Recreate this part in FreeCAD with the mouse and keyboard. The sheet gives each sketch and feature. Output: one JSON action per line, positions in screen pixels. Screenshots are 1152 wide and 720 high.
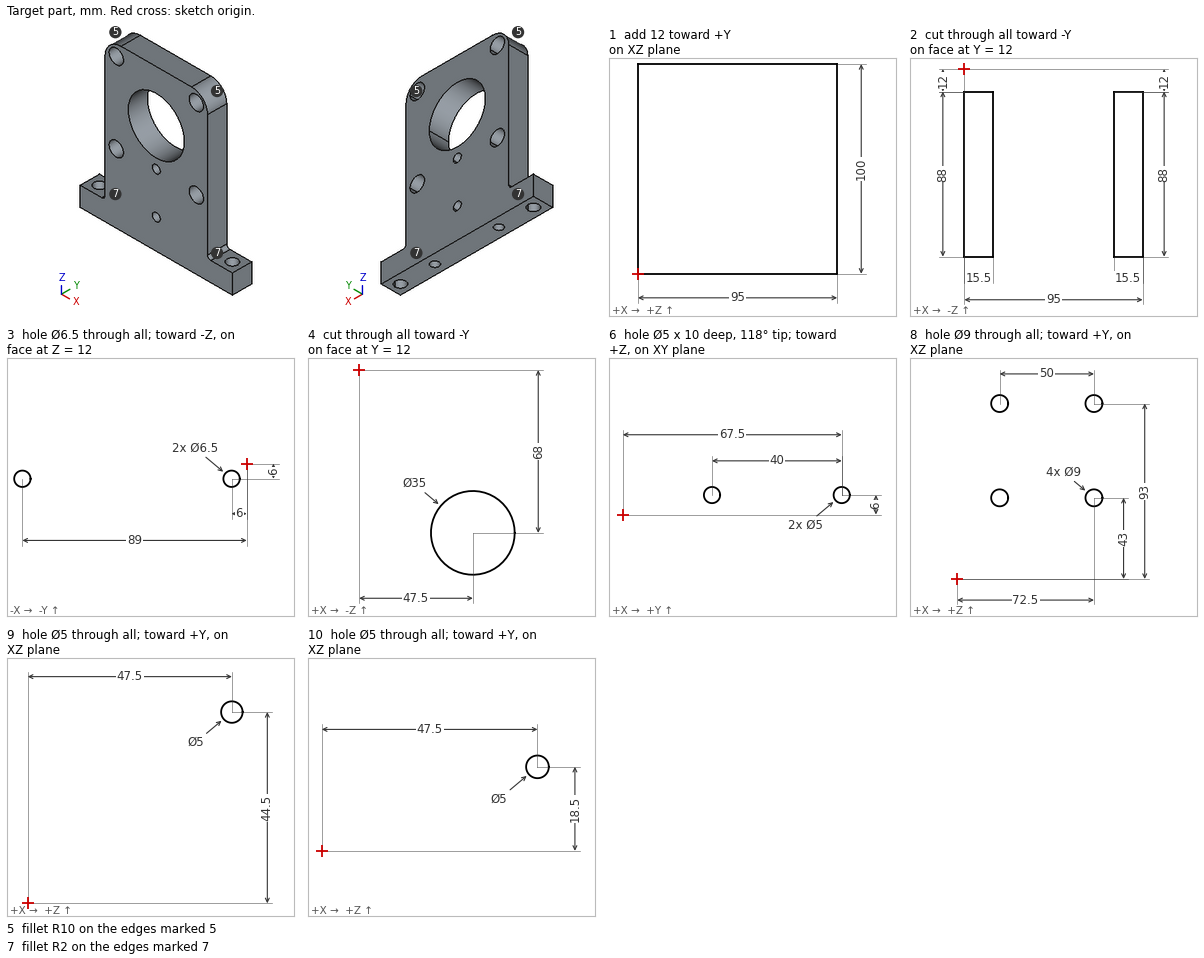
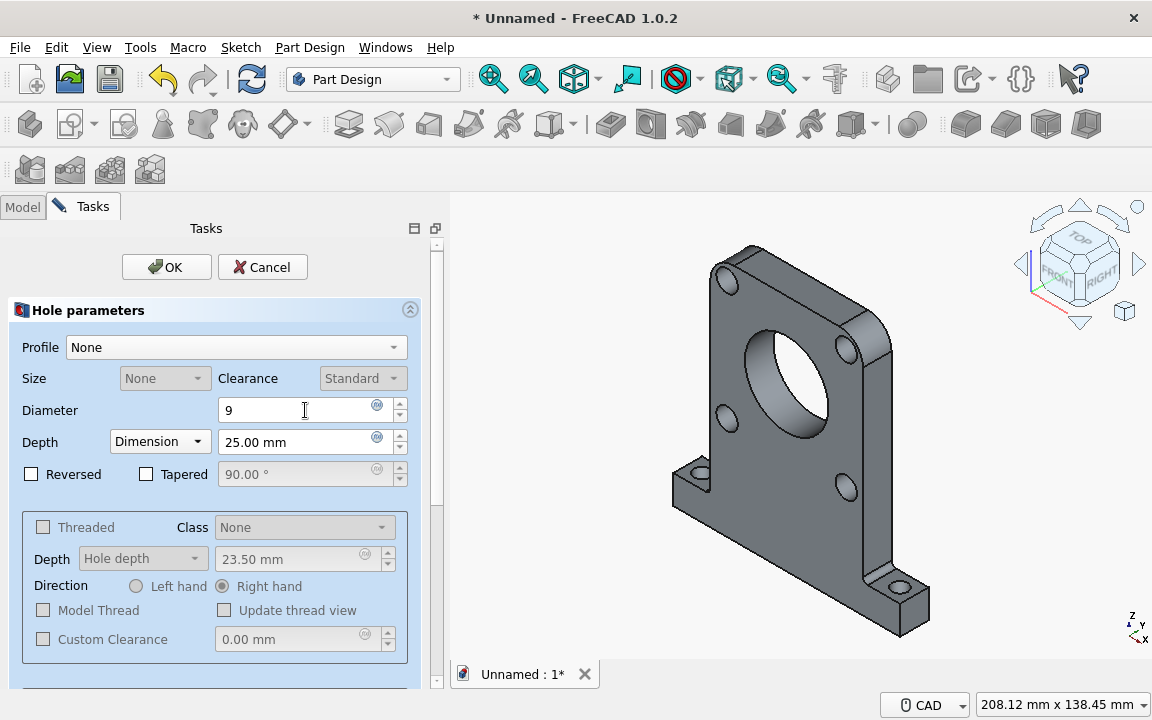
{"action": "left_click", "coordinate": [161, 442]}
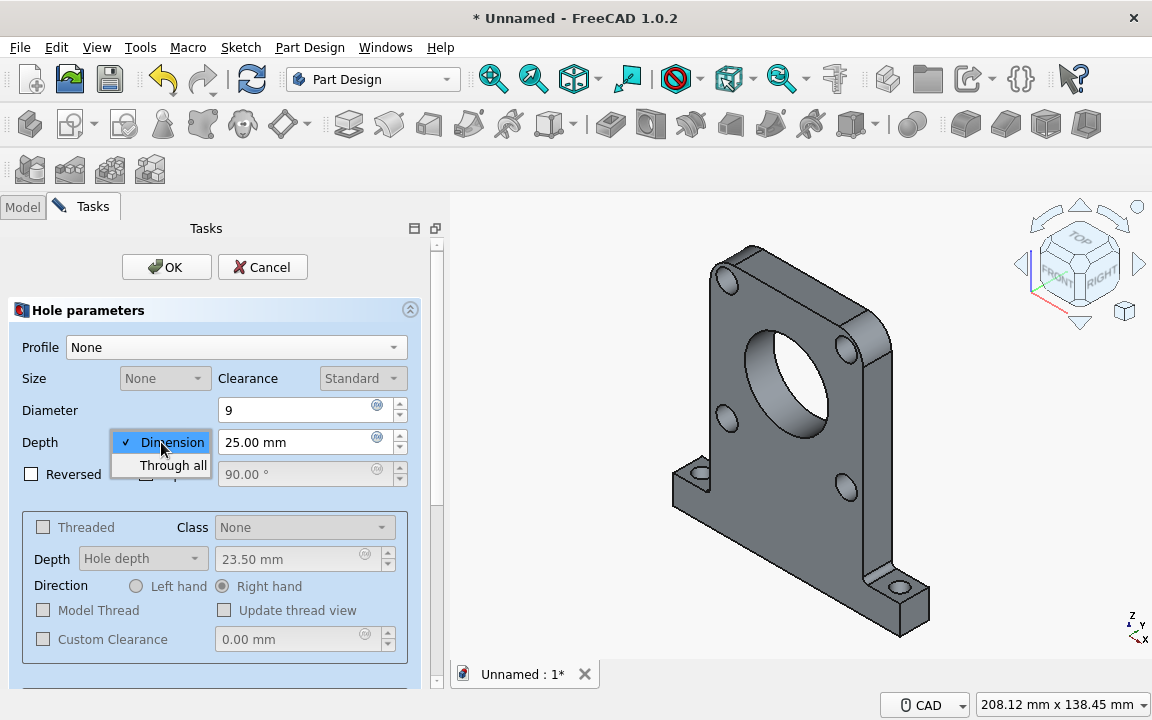
{"action": "left_click", "coordinate": [160, 466]}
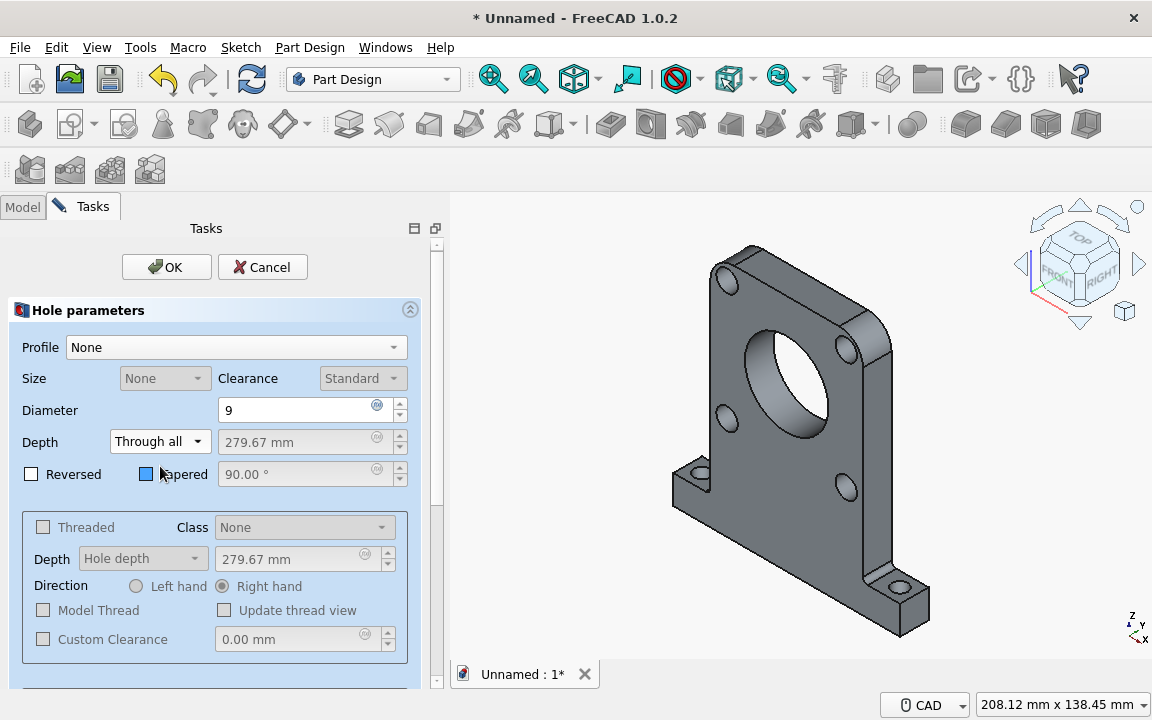
{"action": "left_click", "coordinate": [167, 267]}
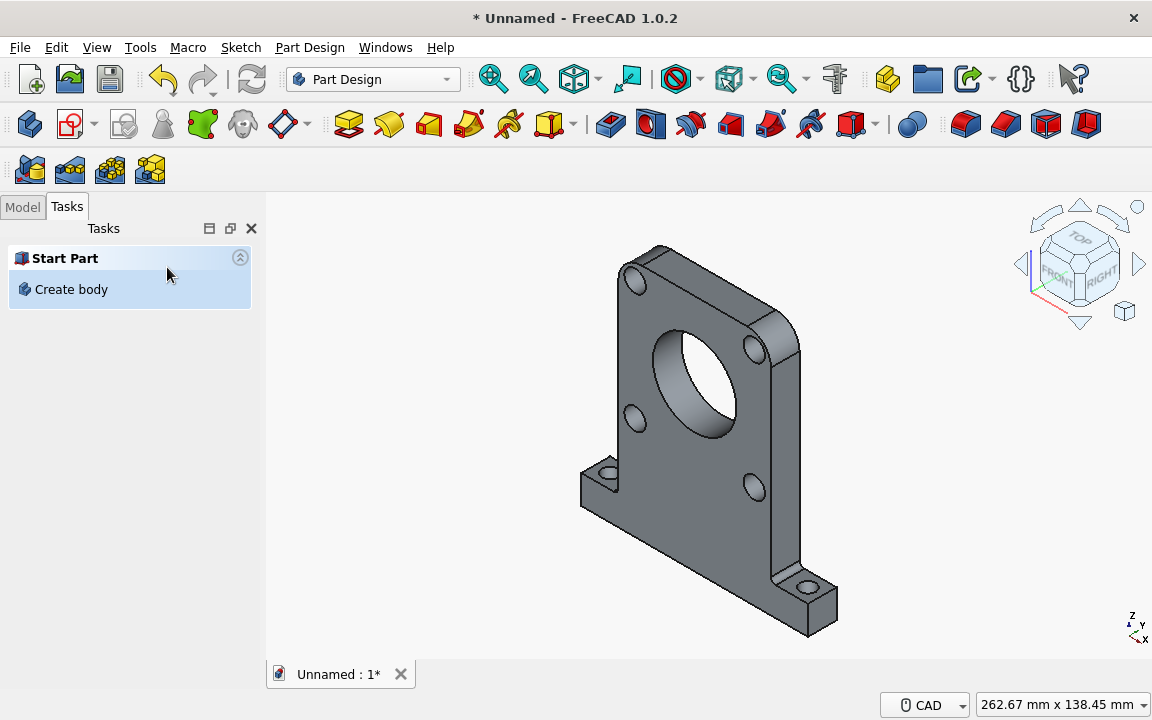
{"action": "left_click", "coordinate": [70, 124]}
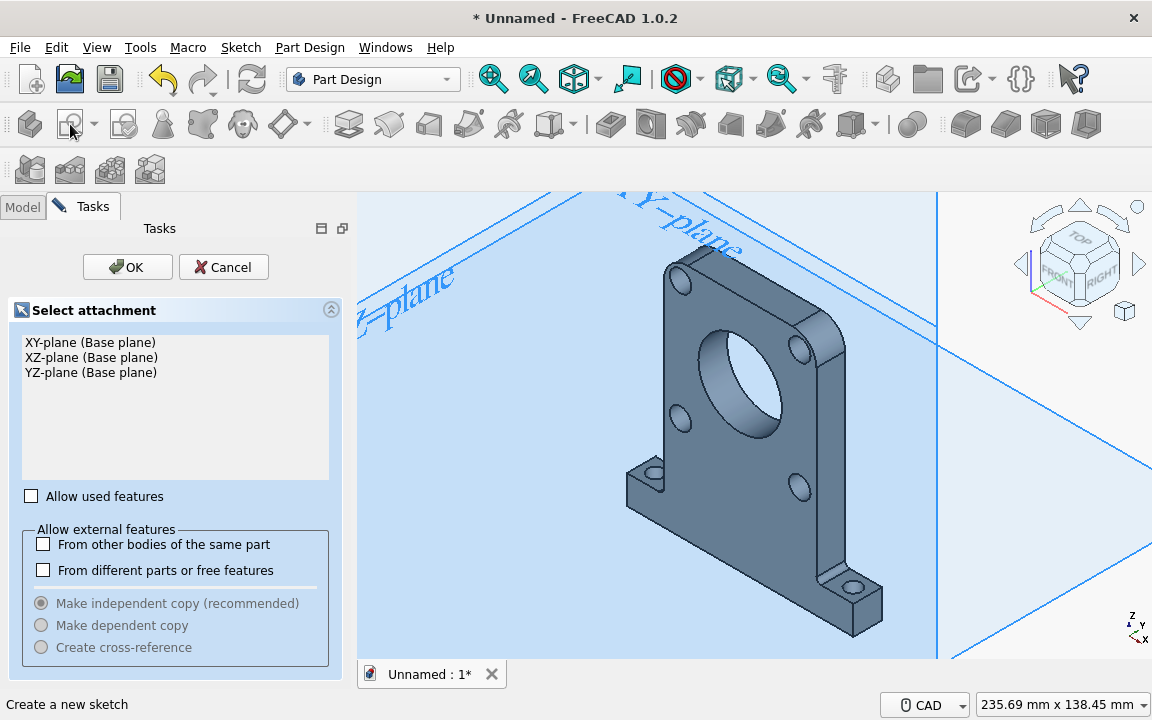
{"action": "left_click", "coordinate": [82, 358]}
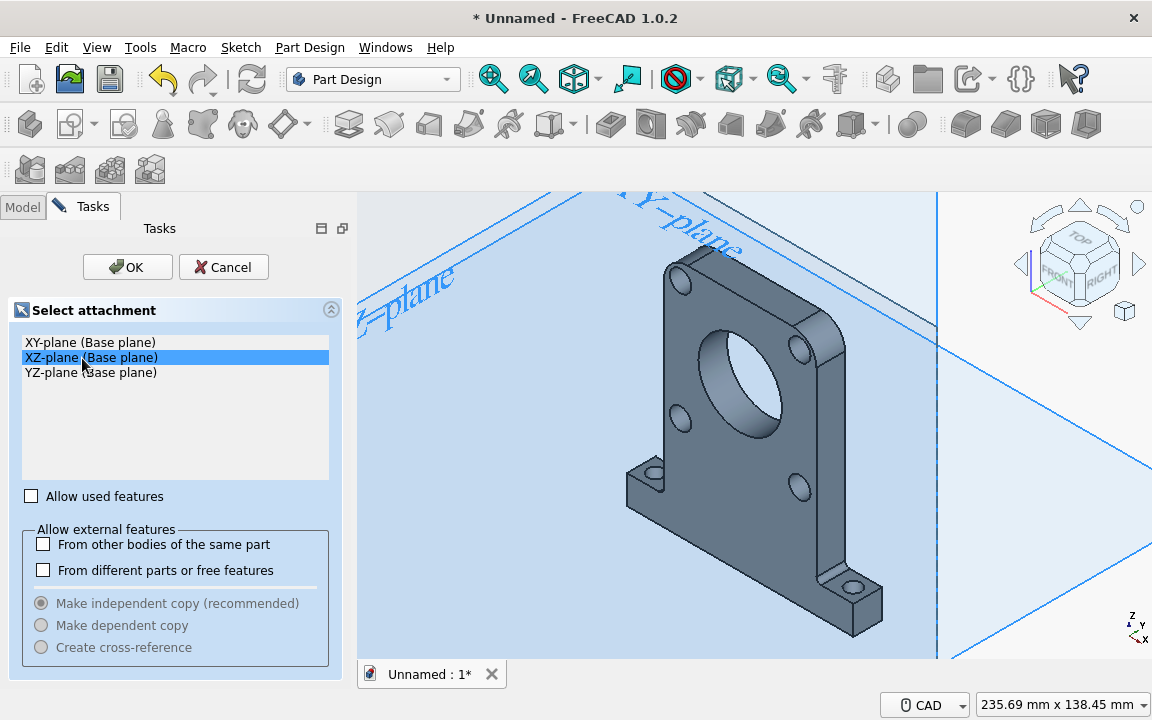
{"action": "left_click", "coordinate": [128, 267]}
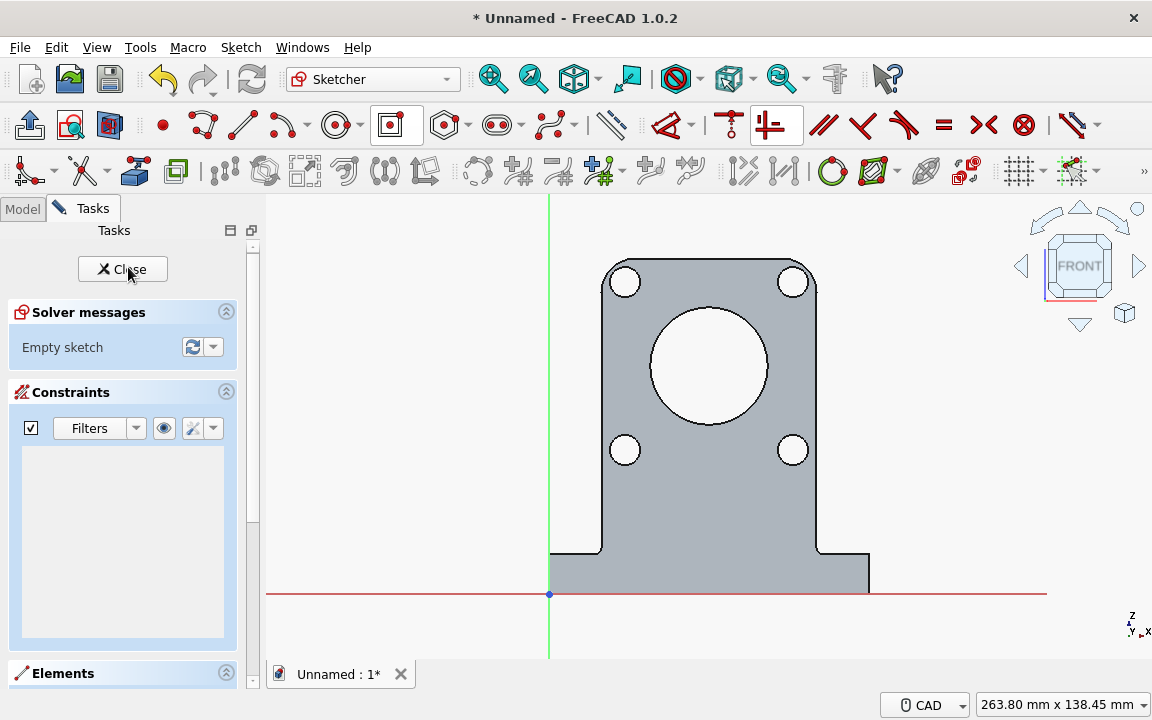
{"action": "scroll", "coordinate": [713, 446], "scroll_direction": "up", "scroll_amount": 14}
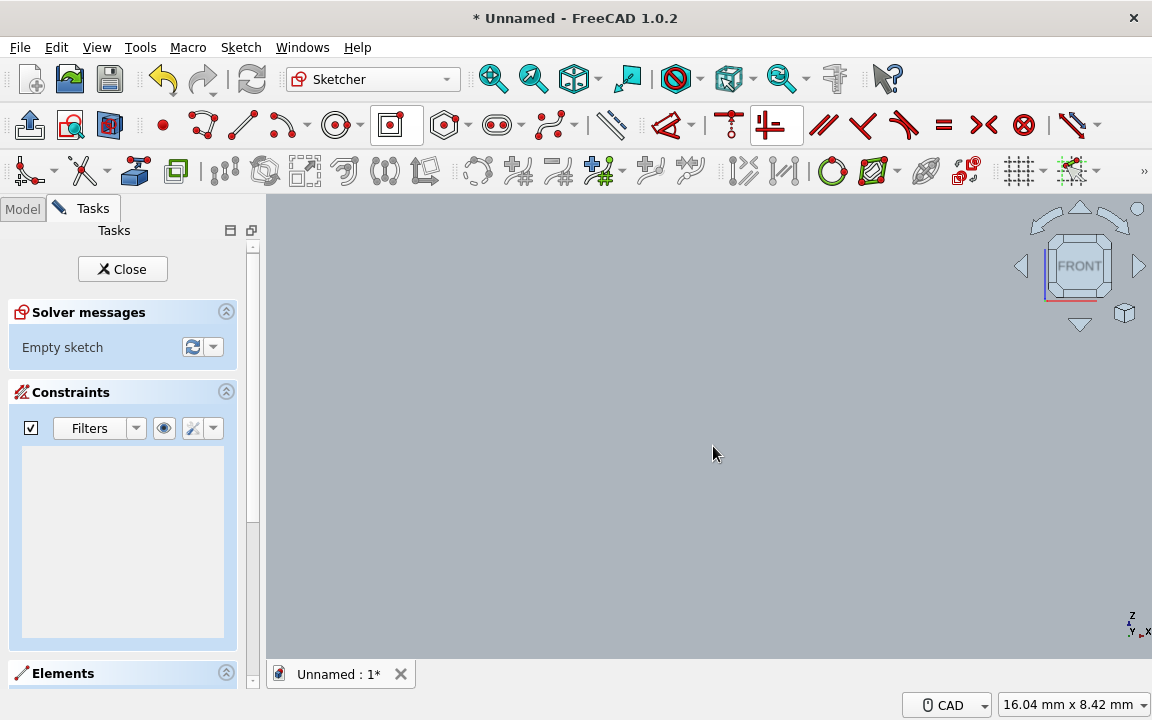
{"action": "left_click", "coordinate": [336, 126]}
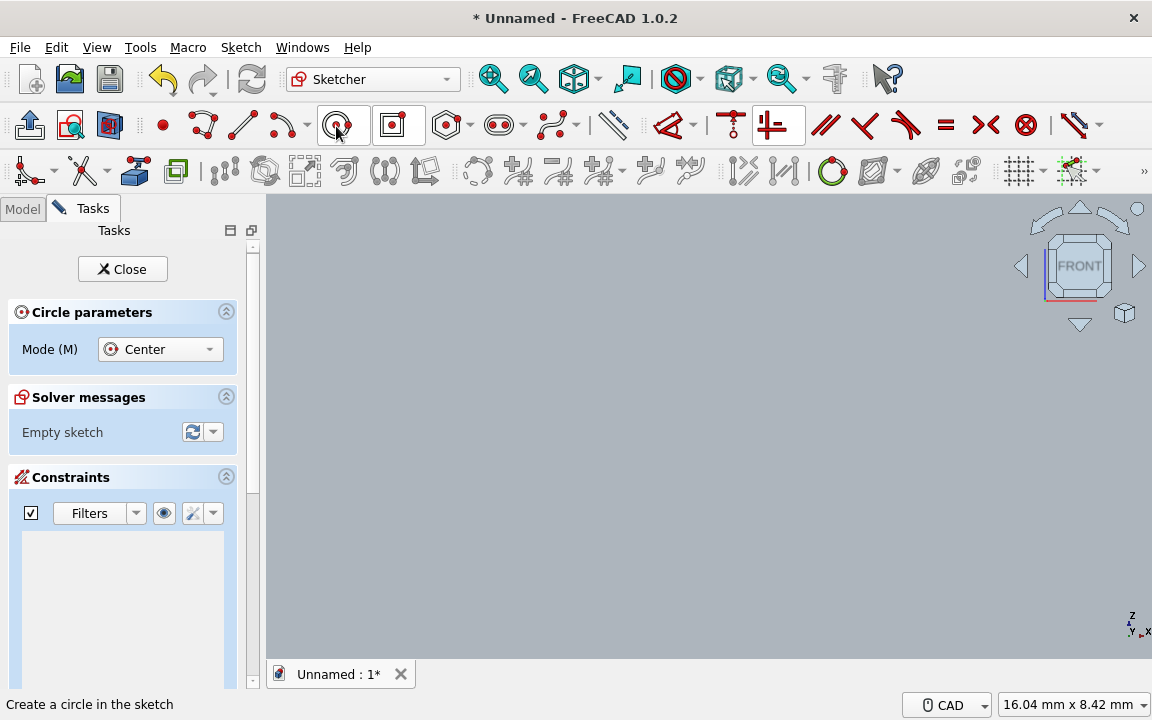
{"action": "left_click", "coordinate": [639, 421]}
{"action": "left_click", "coordinate": [737, 323]}
{"action": "key", "text": "Escape"}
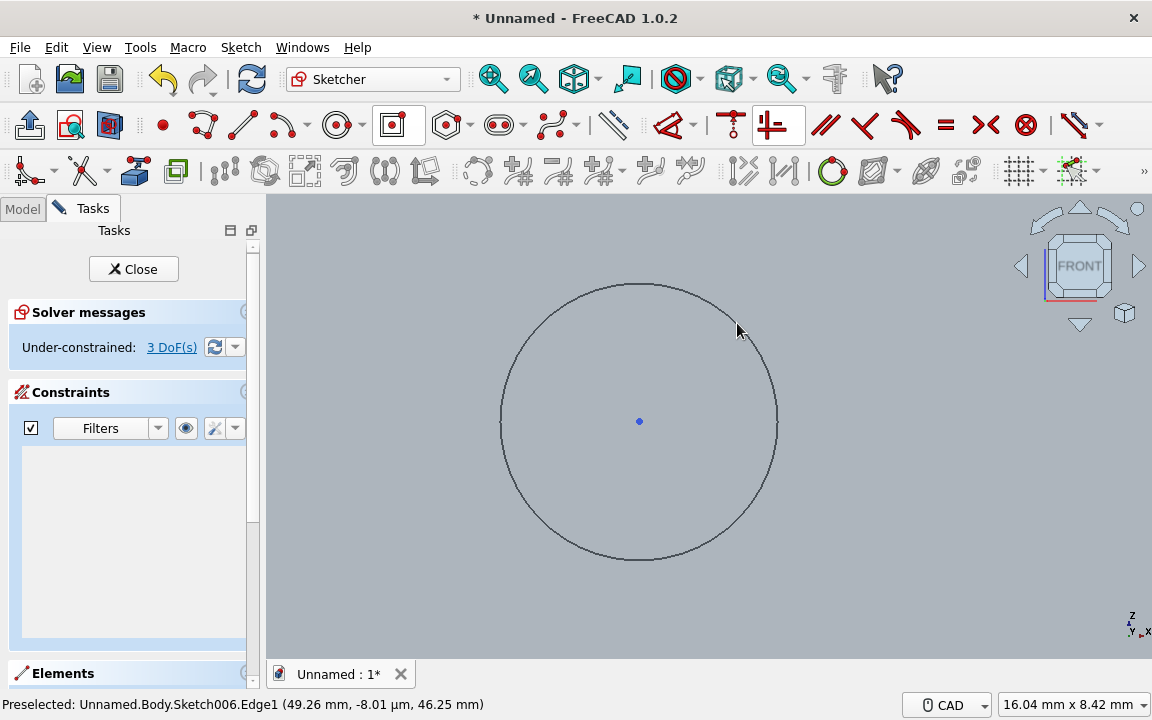
{"action": "left_click", "coordinate": [668, 126]}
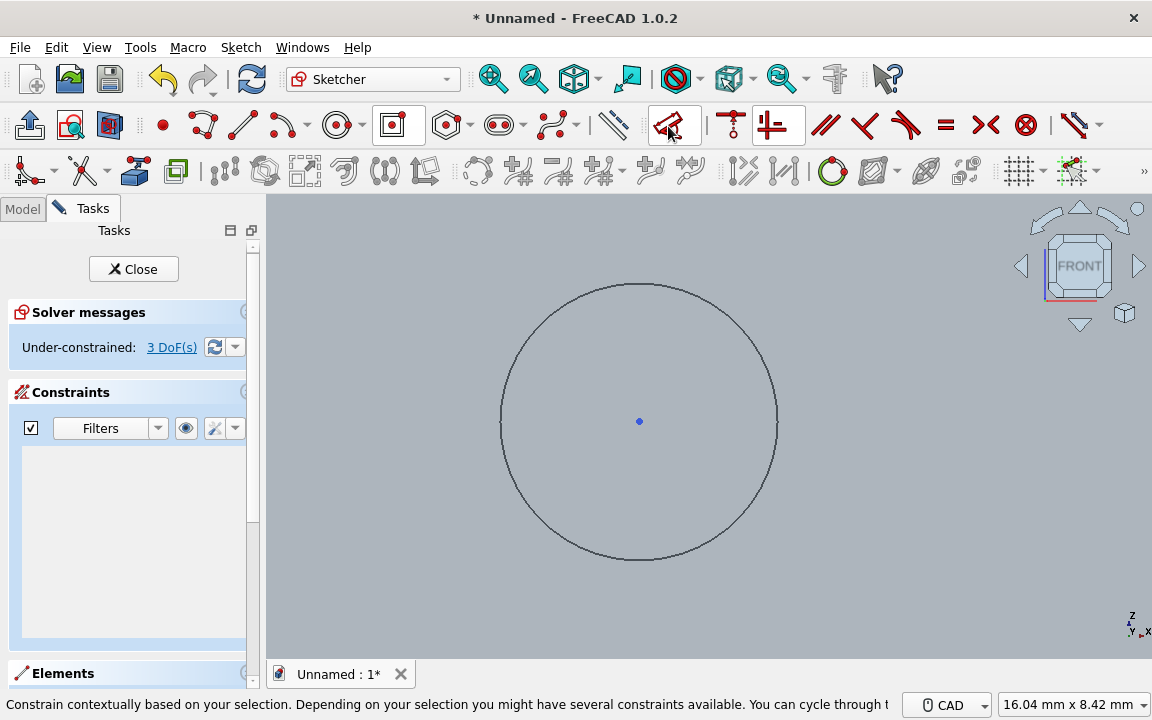
{"action": "left_click", "coordinate": [737, 324]}
{"action": "left_click", "coordinate": [760, 301]}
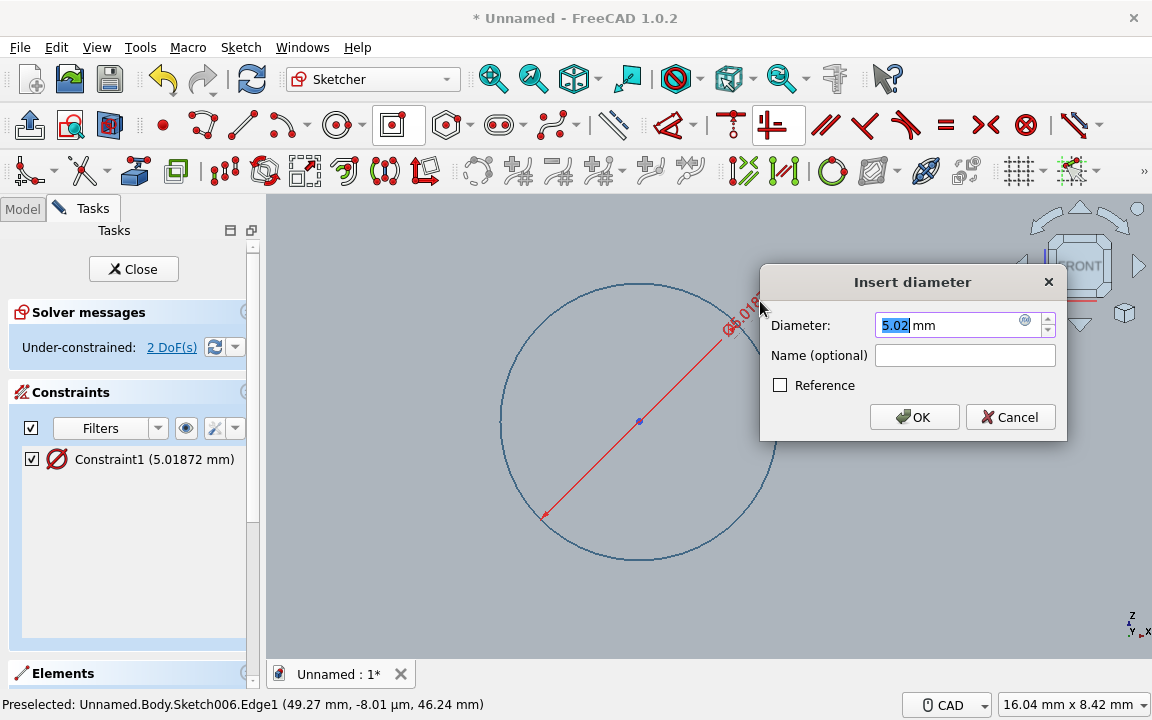
{"action": "type", "text": "5"}
{"action": "key", "text": "Return"}